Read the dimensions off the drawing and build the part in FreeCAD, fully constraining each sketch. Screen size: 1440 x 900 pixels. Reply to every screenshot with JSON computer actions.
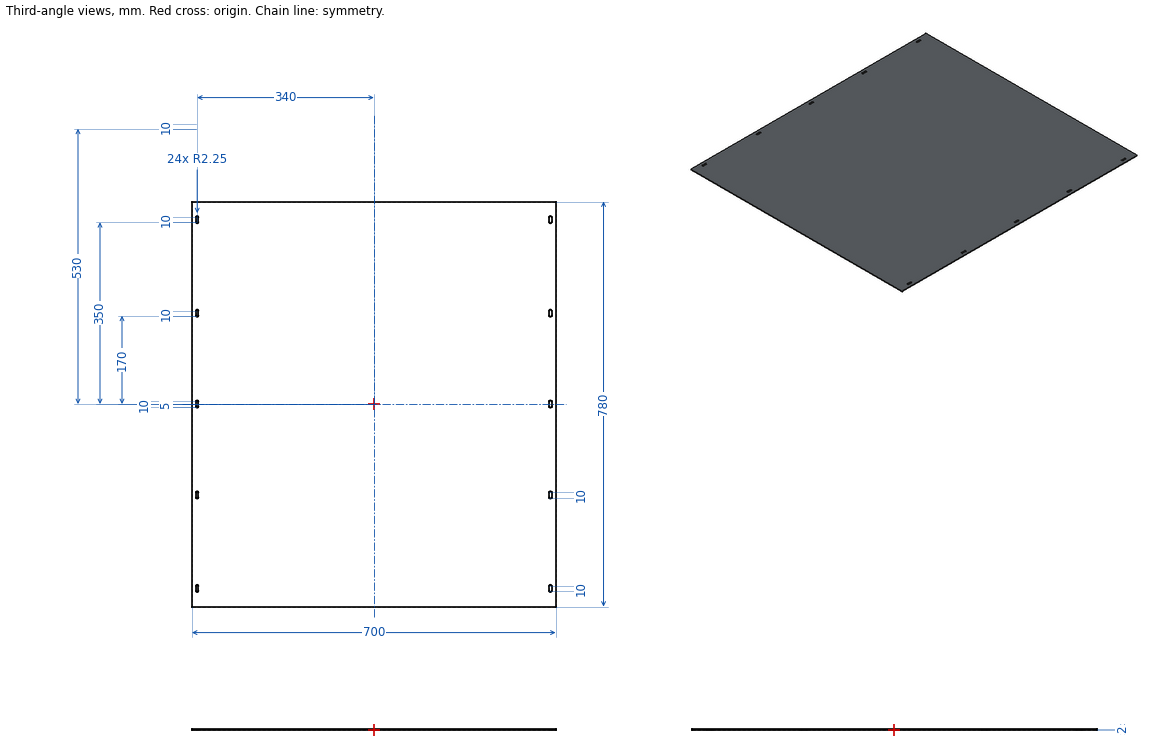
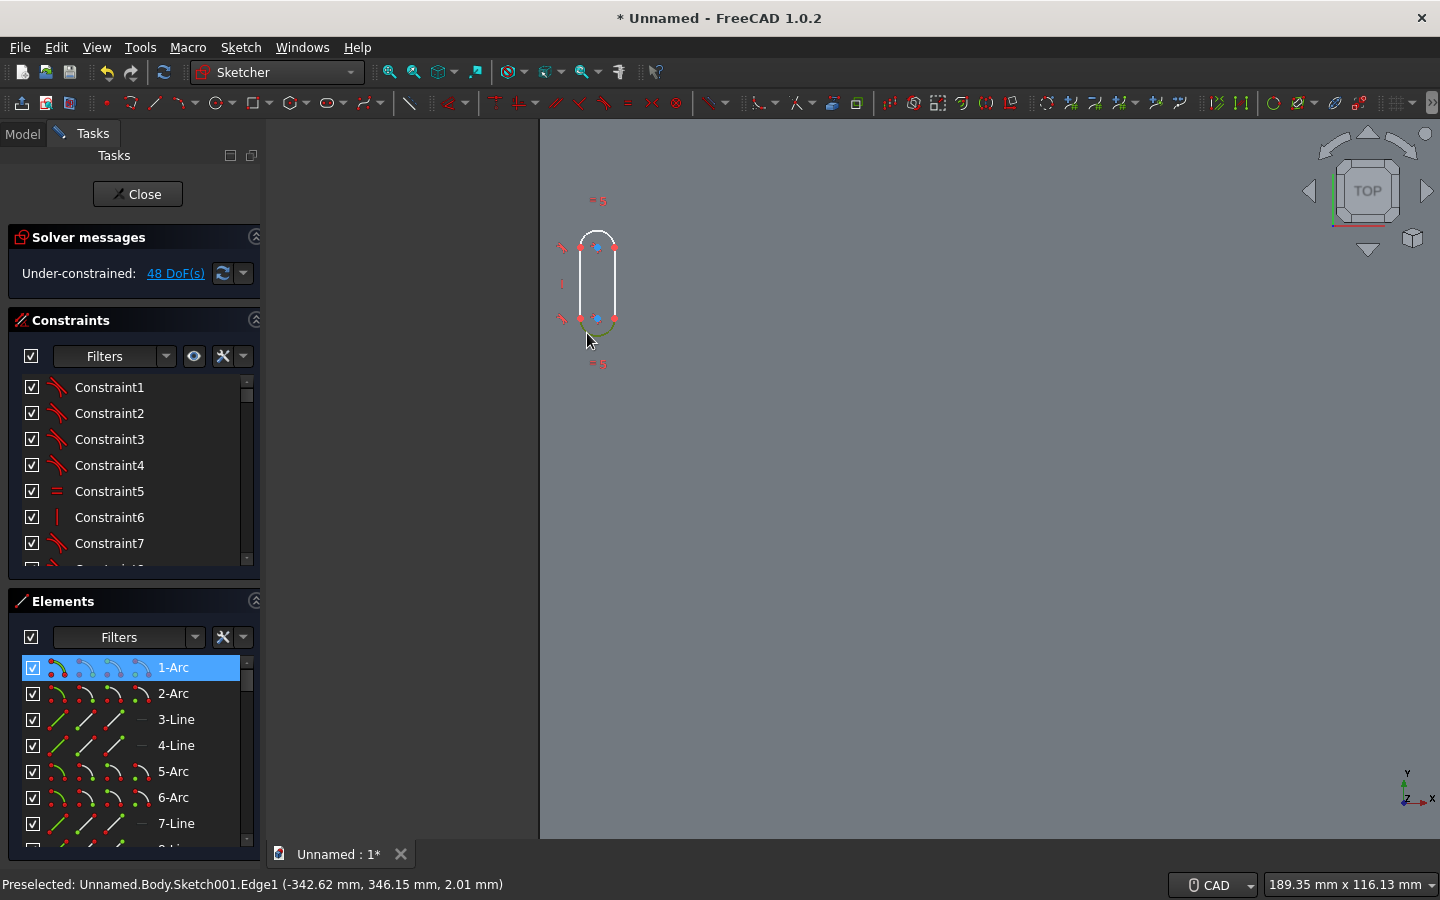
{"action": "scroll", "coordinate": [592, 335], "scroll_direction": "down", "scroll_amount": 12}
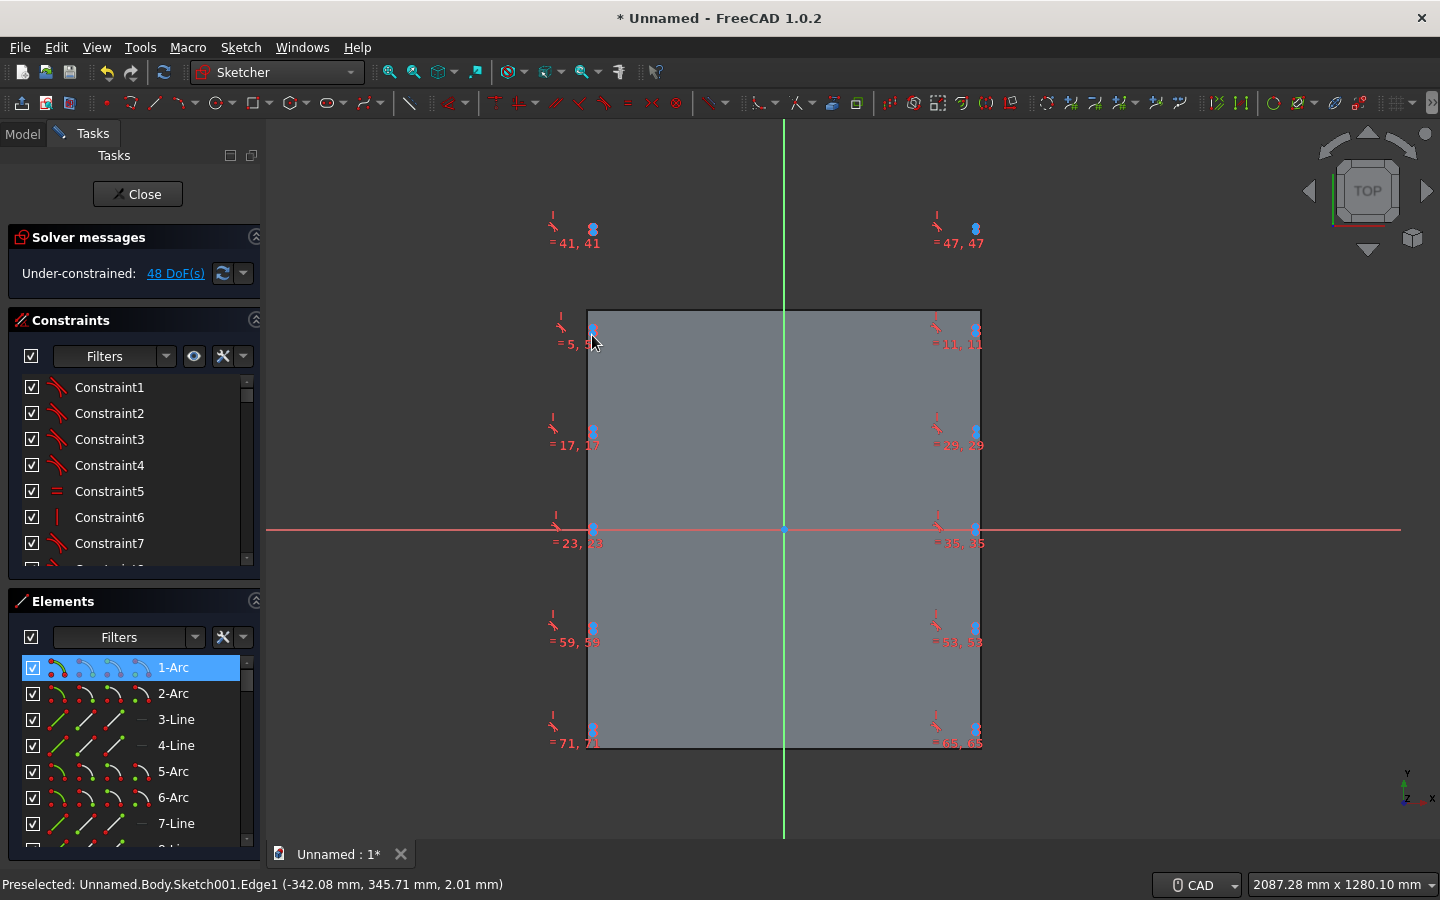
{"action": "scroll", "coordinate": [975, 335], "scroll_direction": "up", "scroll_amount": 12}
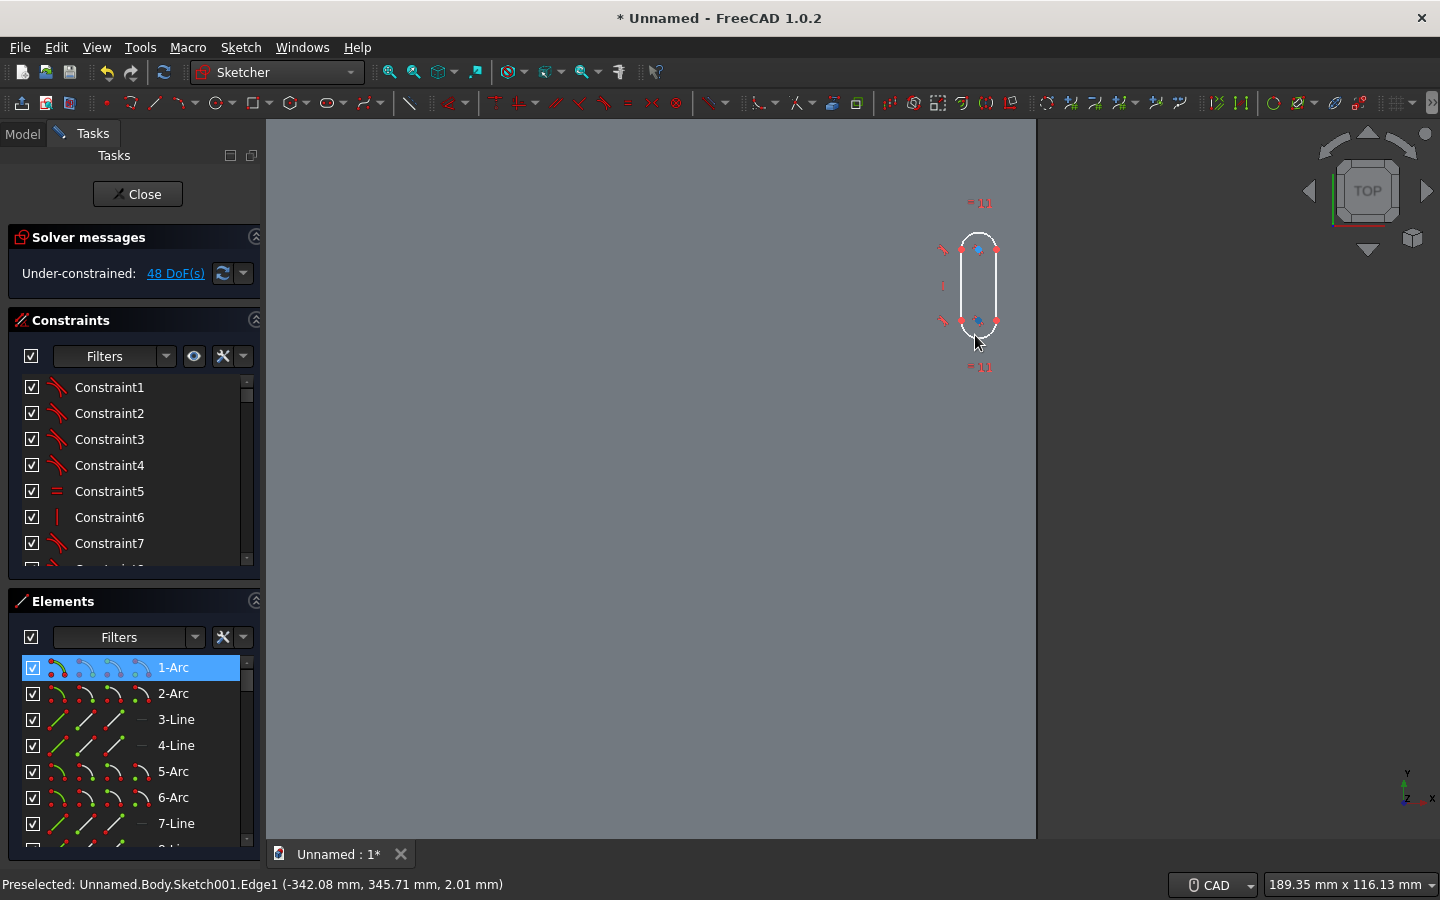
{"action": "left_click", "coordinate": [968, 335]}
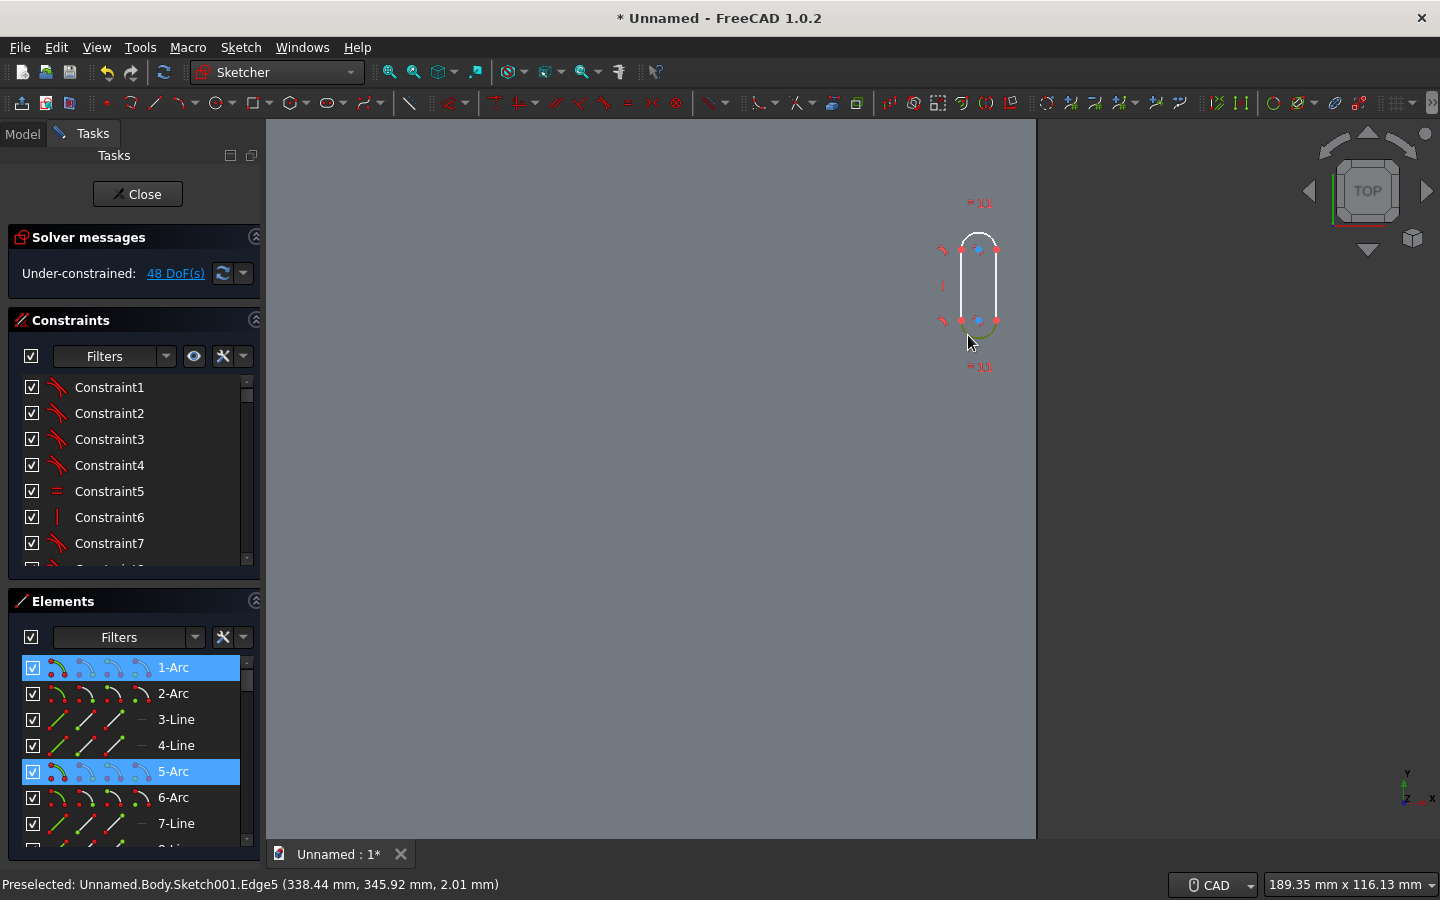
{"action": "scroll", "coordinate": [976, 335], "scroll_direction": "down", "scroll_amount": 12}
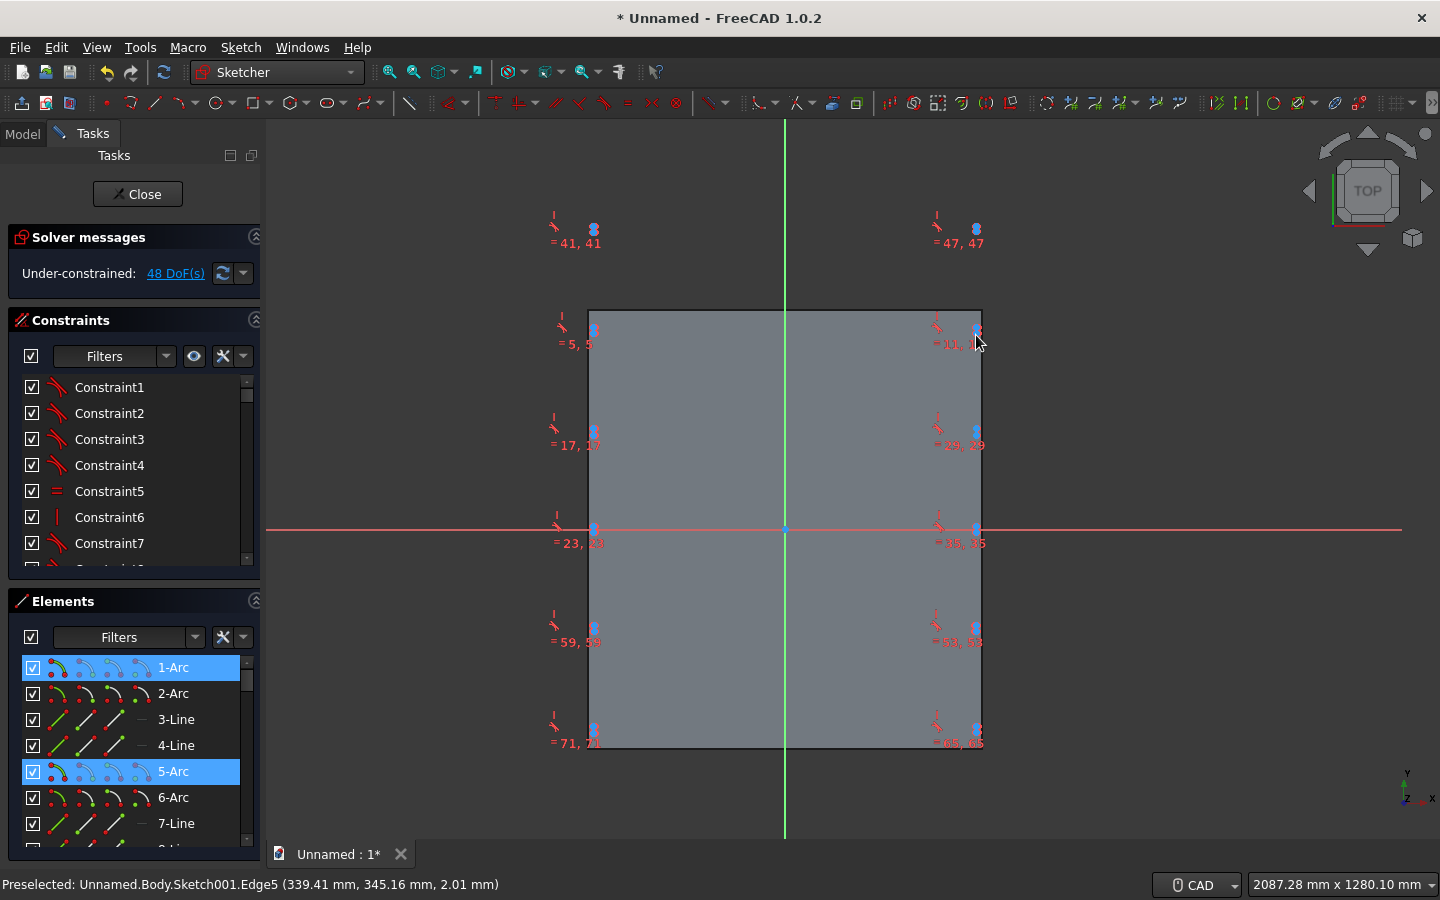
{"action": "scroll", "coordinate": [593, 436], "scroll_direction": "up", "scroll_amount": 13}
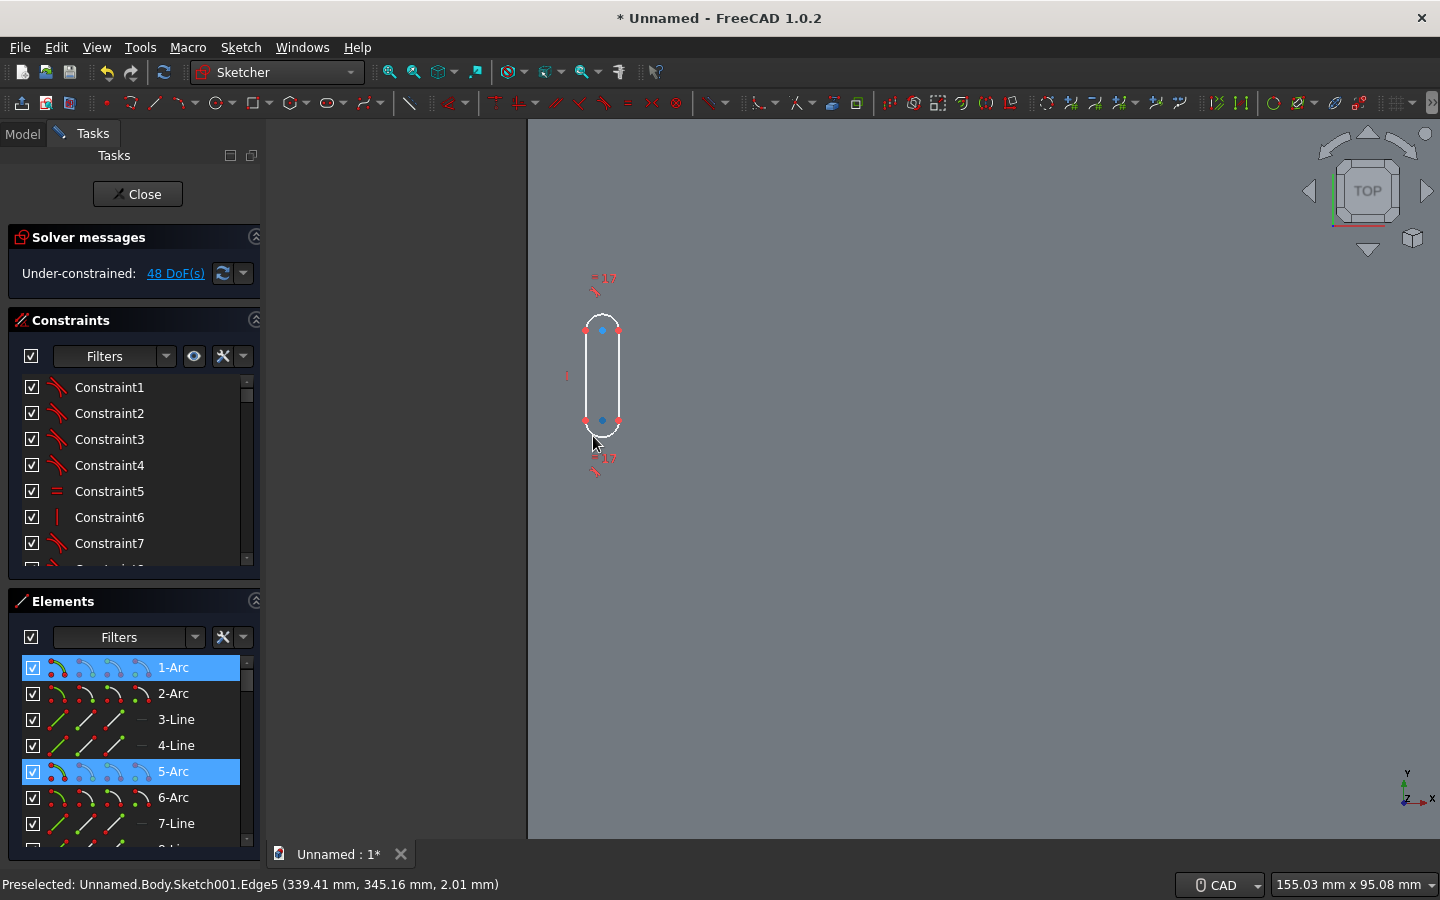
{"action": "left_click", "coordinate": [593, 434]}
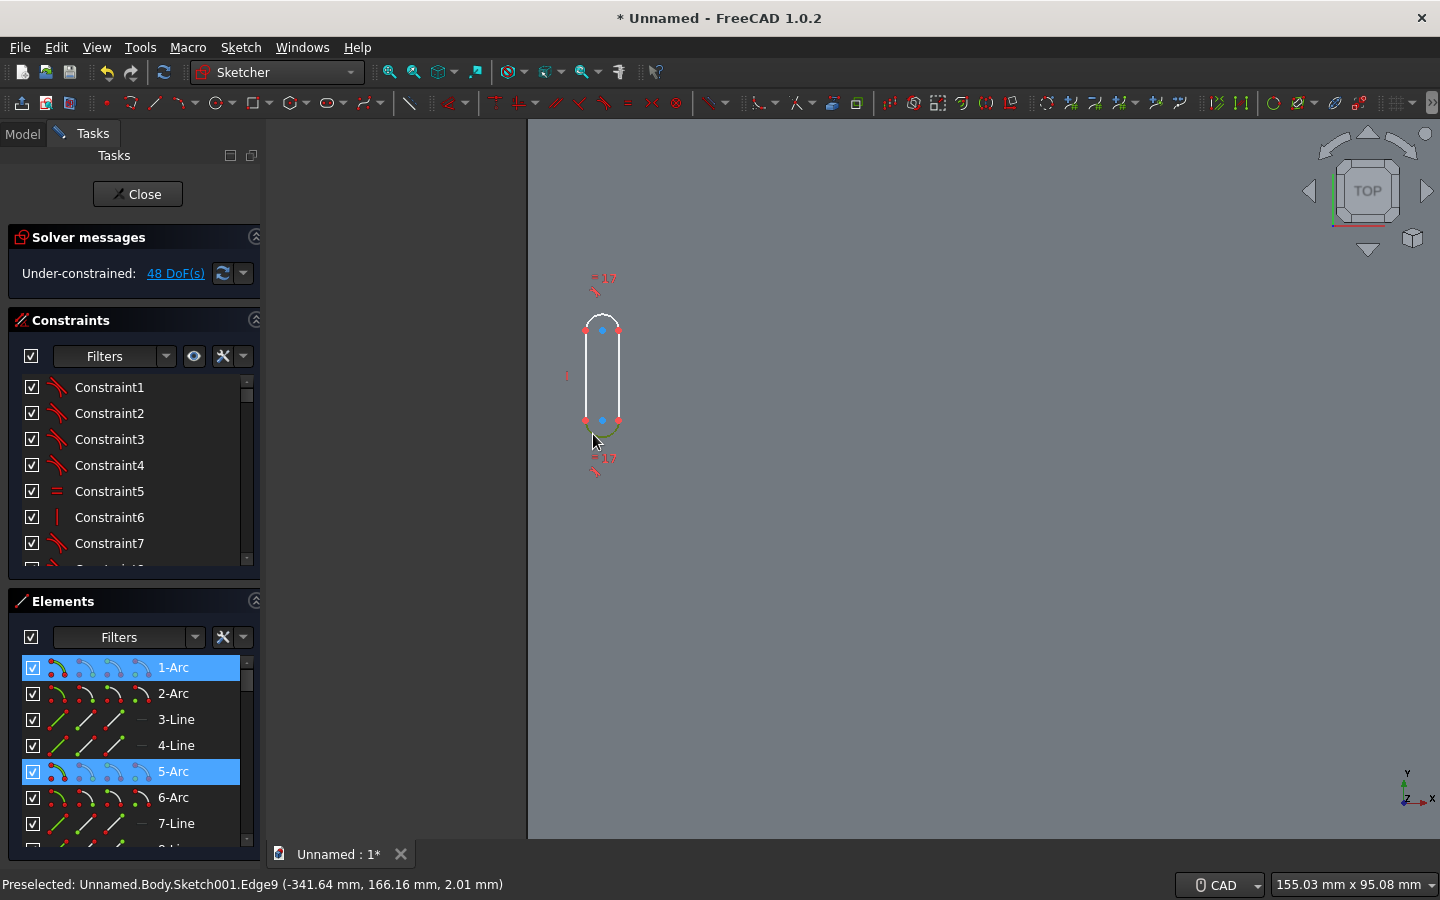
{"action": "scroll", "coordinate": [592, 437], "scroll_direction": "down", "scroll_amount": 13}